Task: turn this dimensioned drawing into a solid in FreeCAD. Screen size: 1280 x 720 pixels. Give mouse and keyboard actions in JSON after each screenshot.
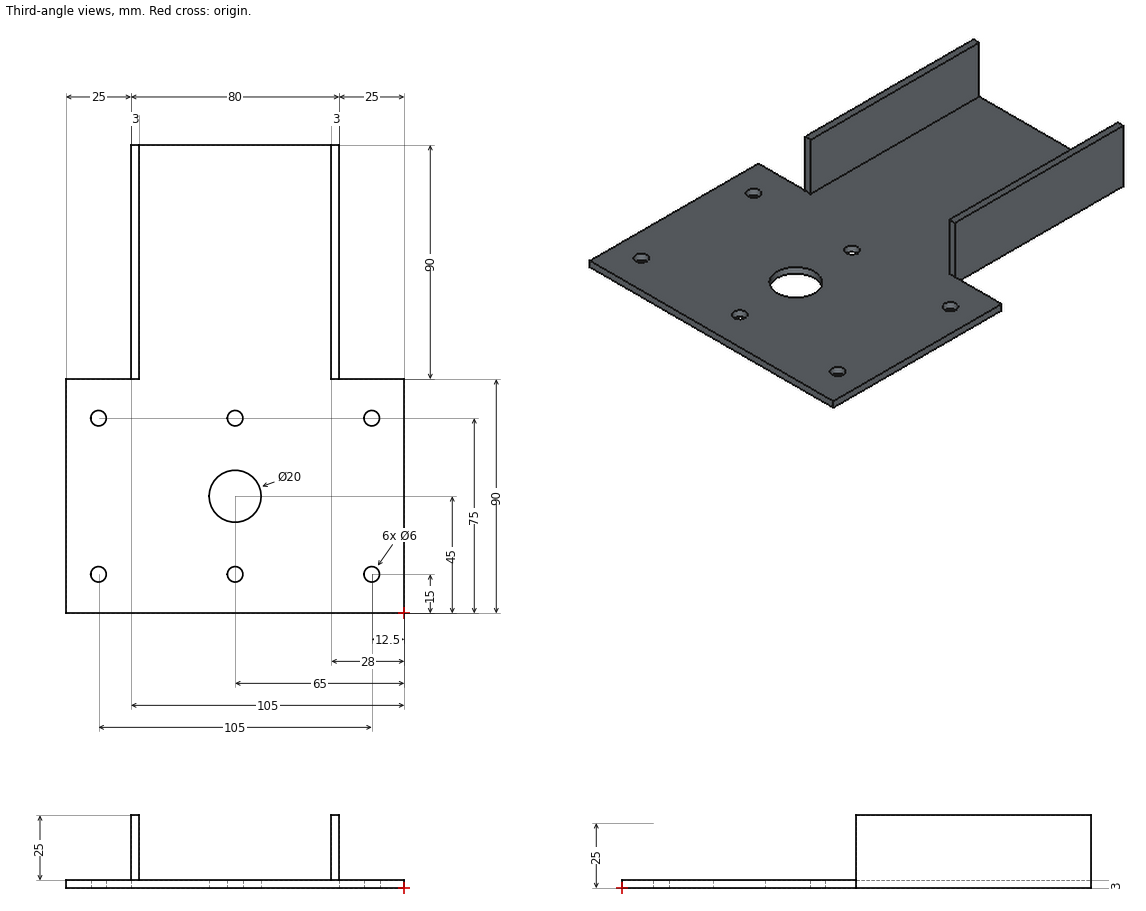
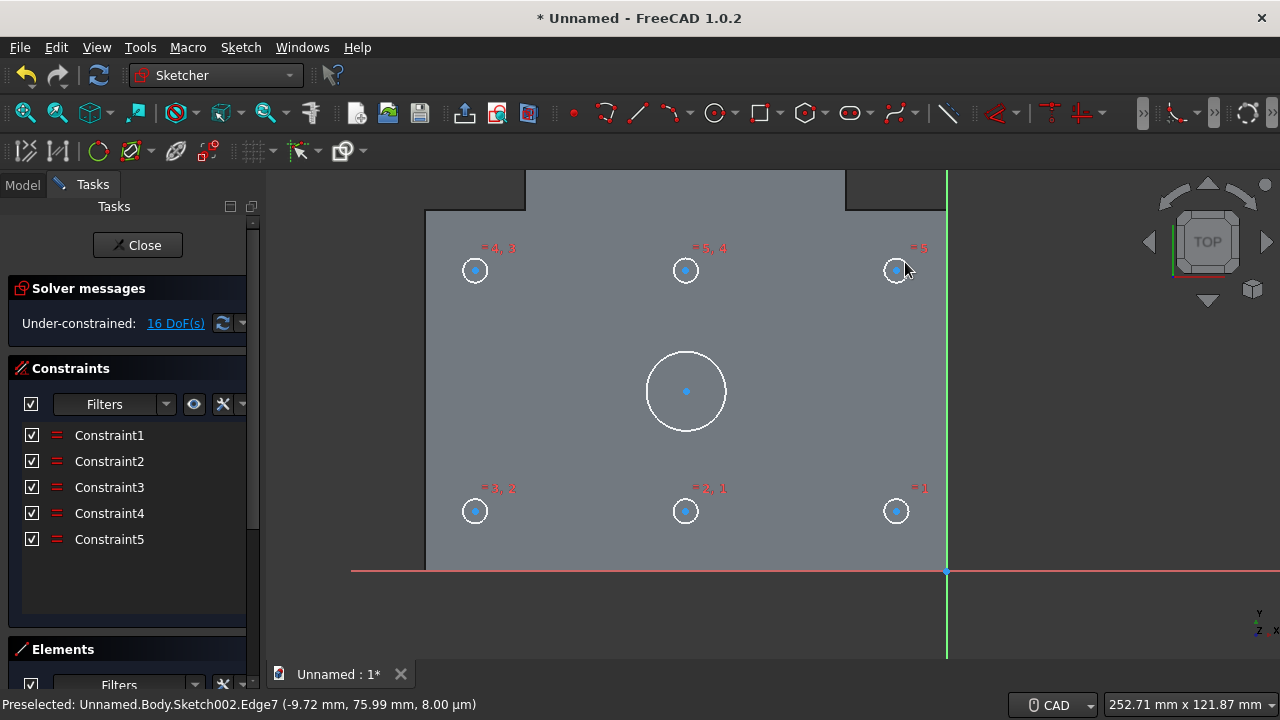
{"action": "left_click", "coordinate": [996, 114]}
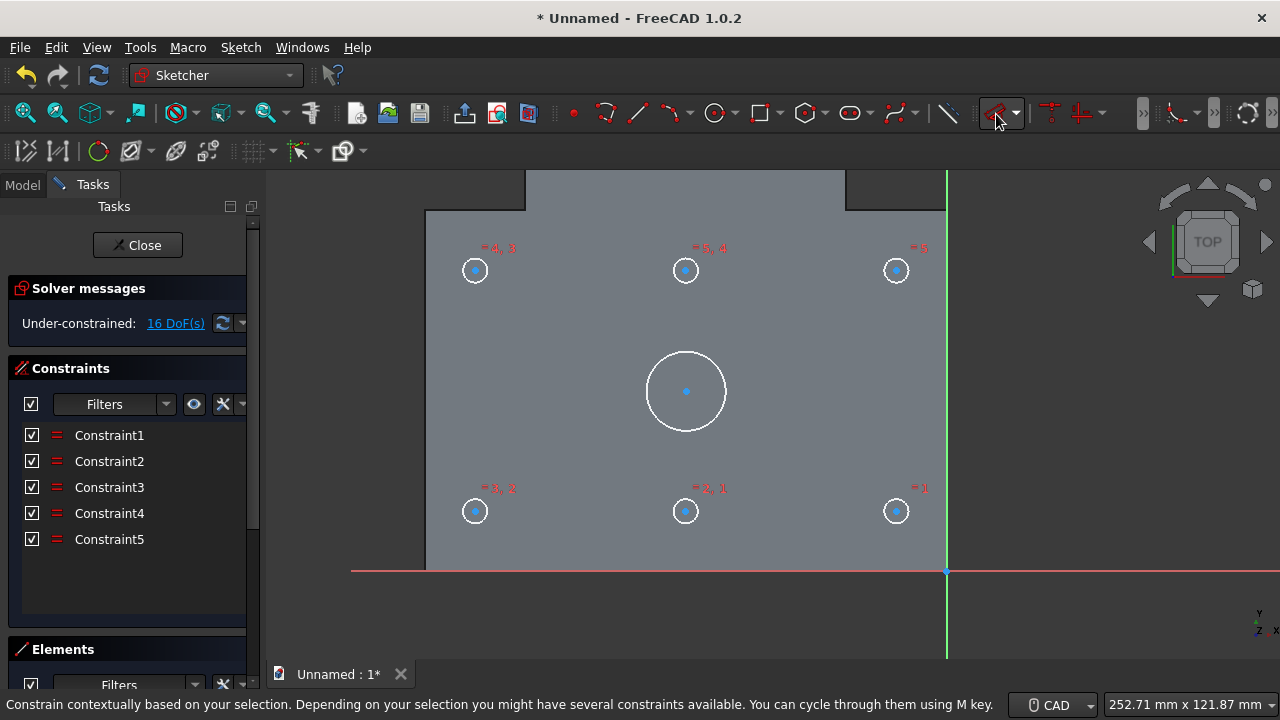
{"action": "left_click", "coordinate": [714, 363]}
{"action": "left_click", "coordinate": [736, 340]}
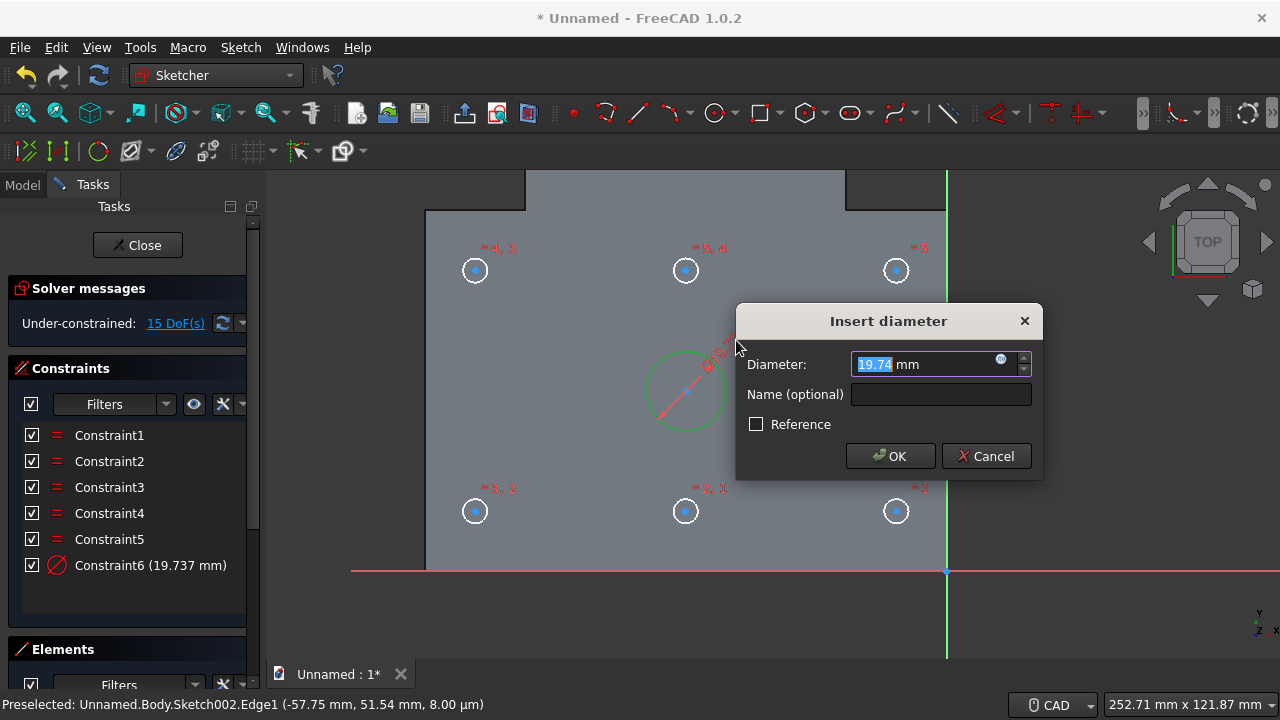
{"action": "type", "text": "20"}
{"action": "key", "text": "Return"}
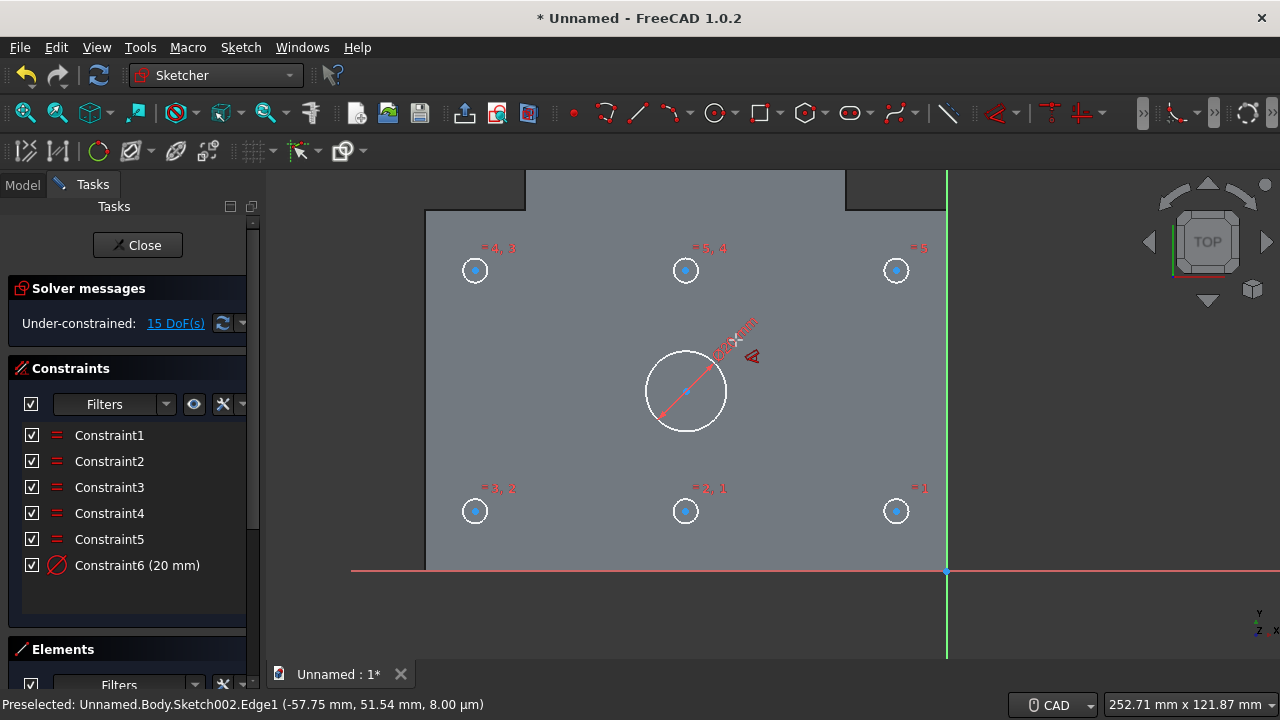
{"action": "scroll", "coordinate": [905, 503], "scroll_direction": "up", "scroll_amount": 3}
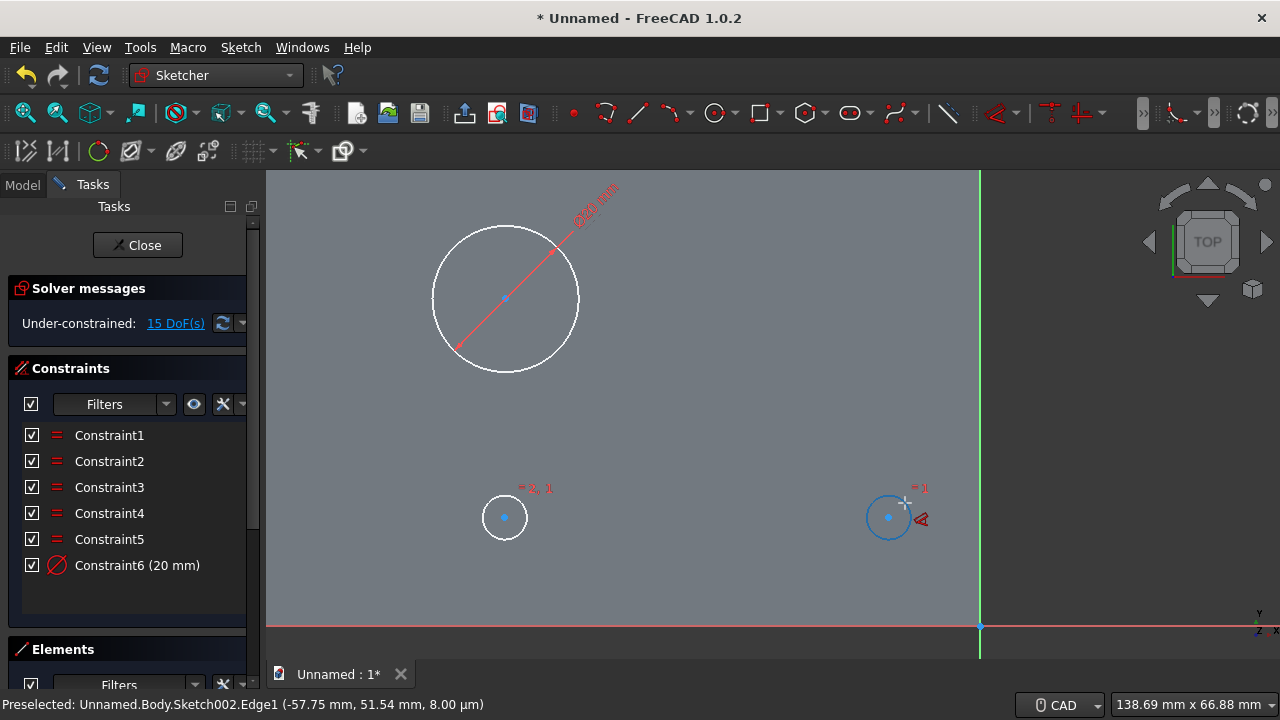
{"action": "left_click", "coordinate": [904, 502]}
{"action": "left_click", "coordinate": [926, 479]}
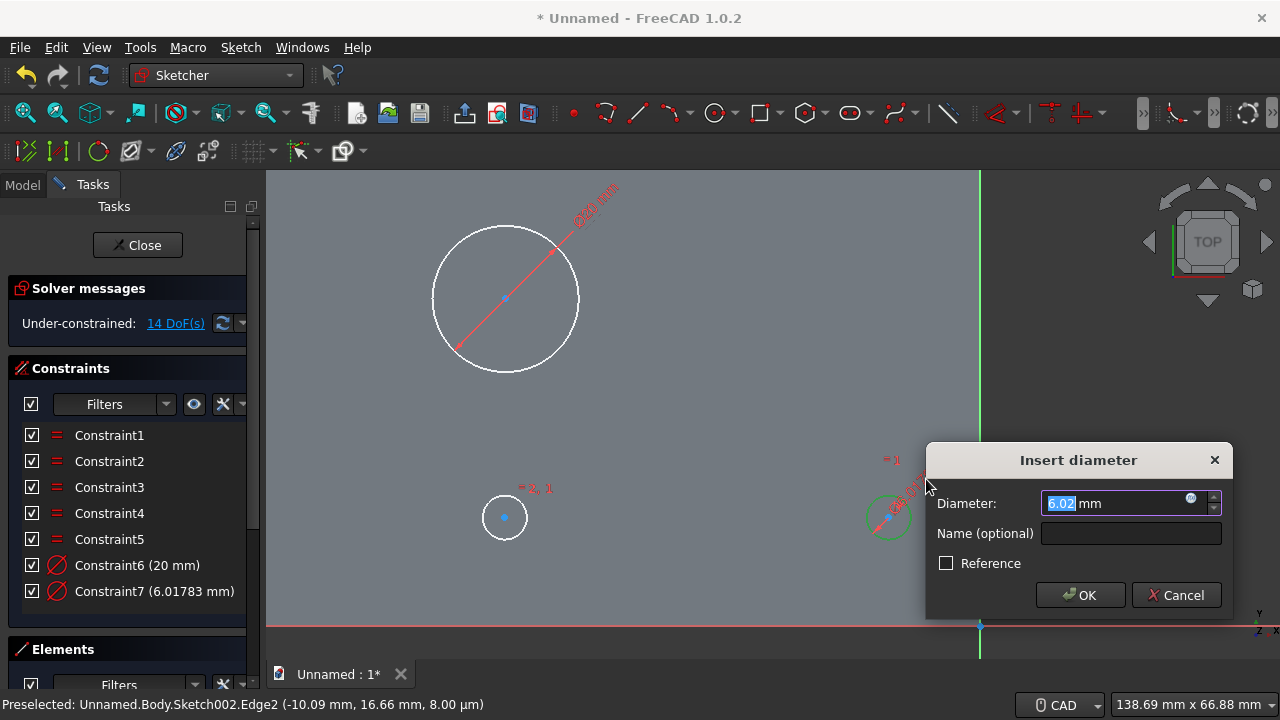
{"action": "type", "text": "6"}
{"action": "key", "text": "Return"}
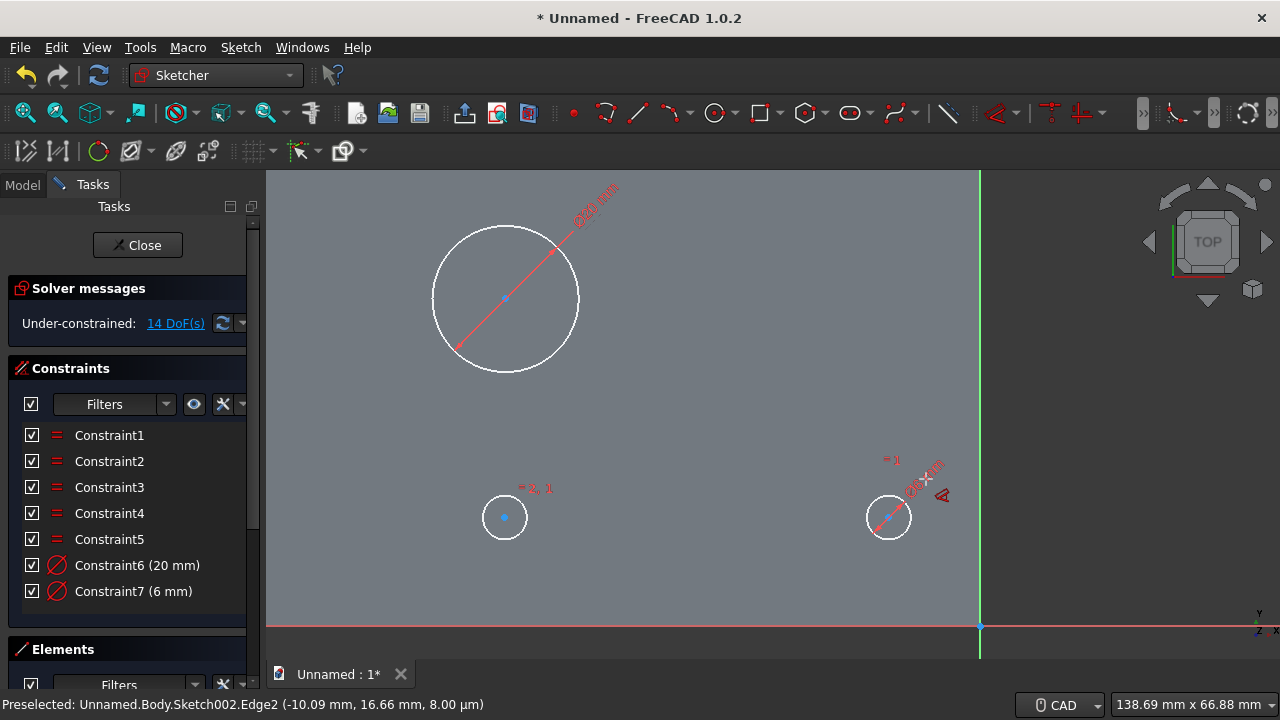
{"action": "left_click", "coordinate": [506, 299]}
{"action": "left_click", "coordinate": [743, 265]}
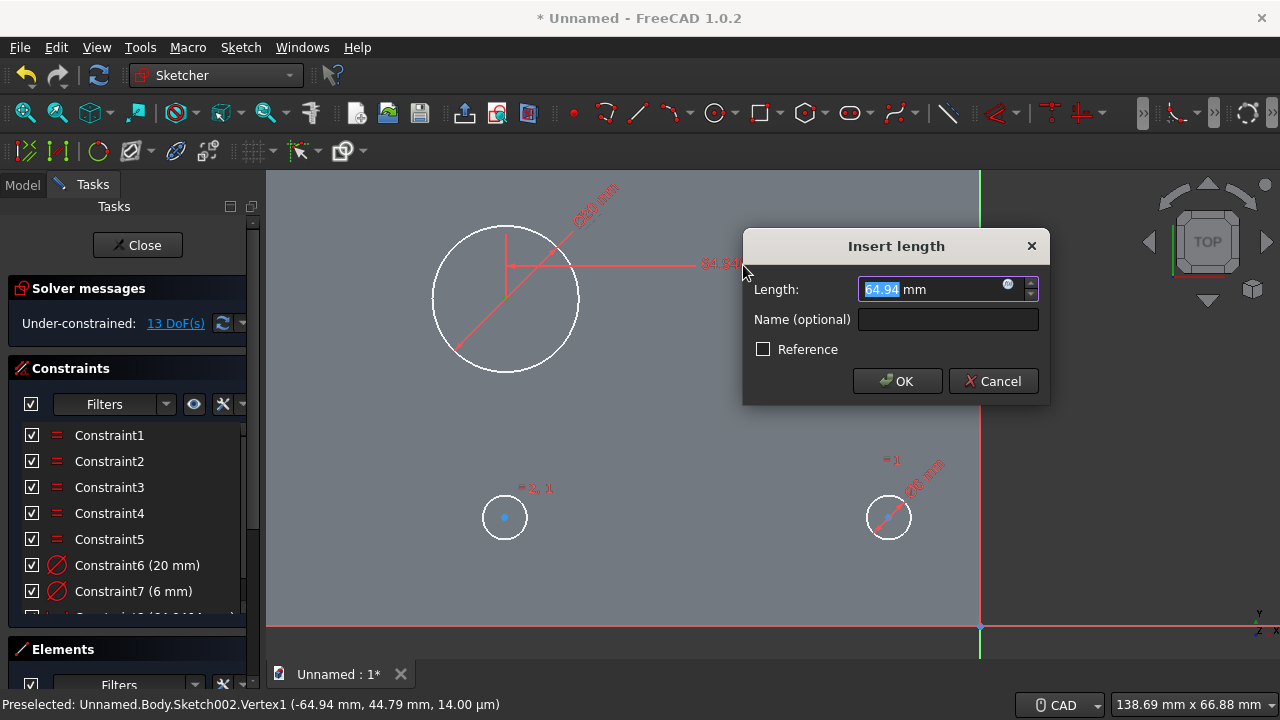
{"action": "type", "text": "65"}
{"action": "key", "text": "Return"}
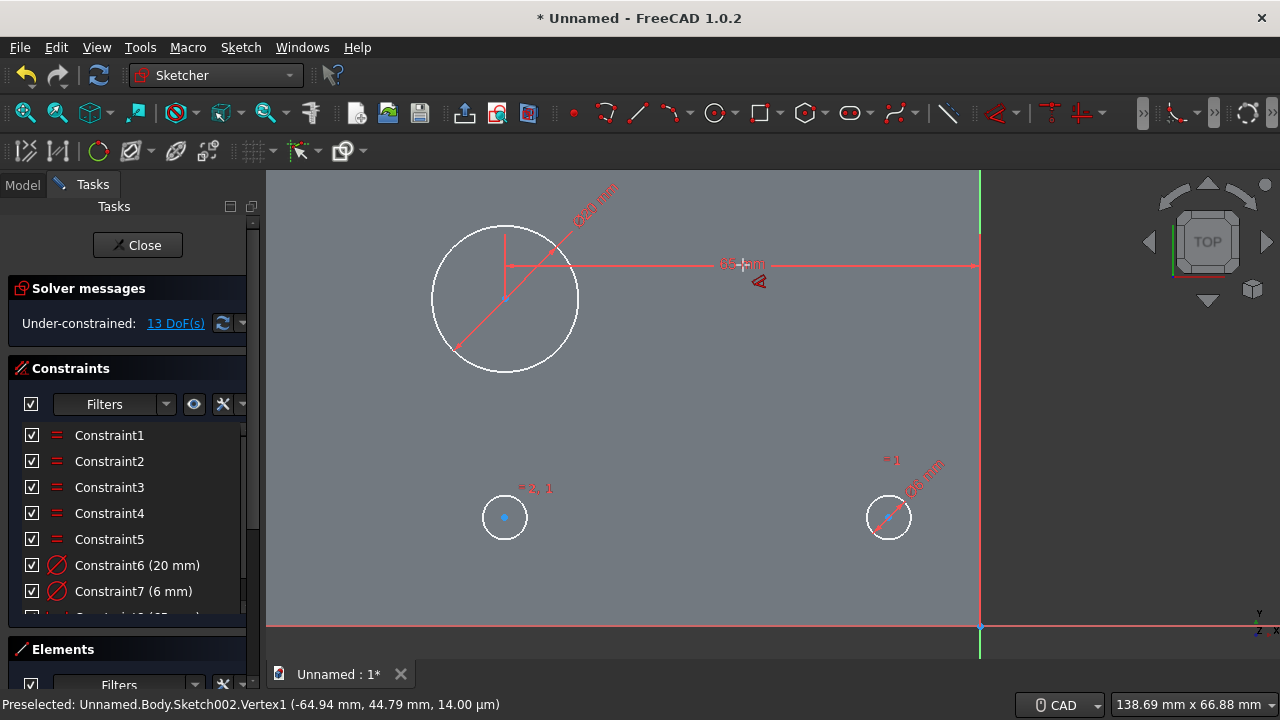
{"action": "left_click", "coordinate": [505, 299]}
{"action": "left_click", "coordinate": [1014, 463]}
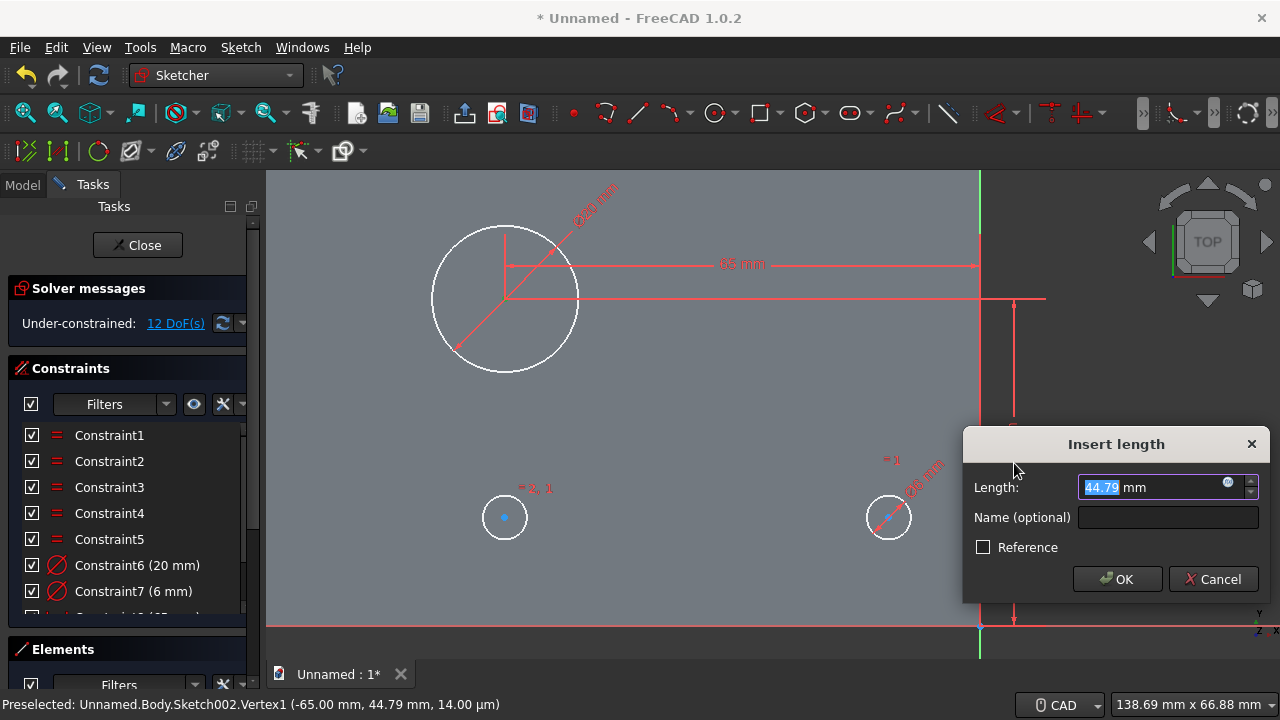
{"action": "type", "text": "45"}
{"action": "key", "text": "Return"}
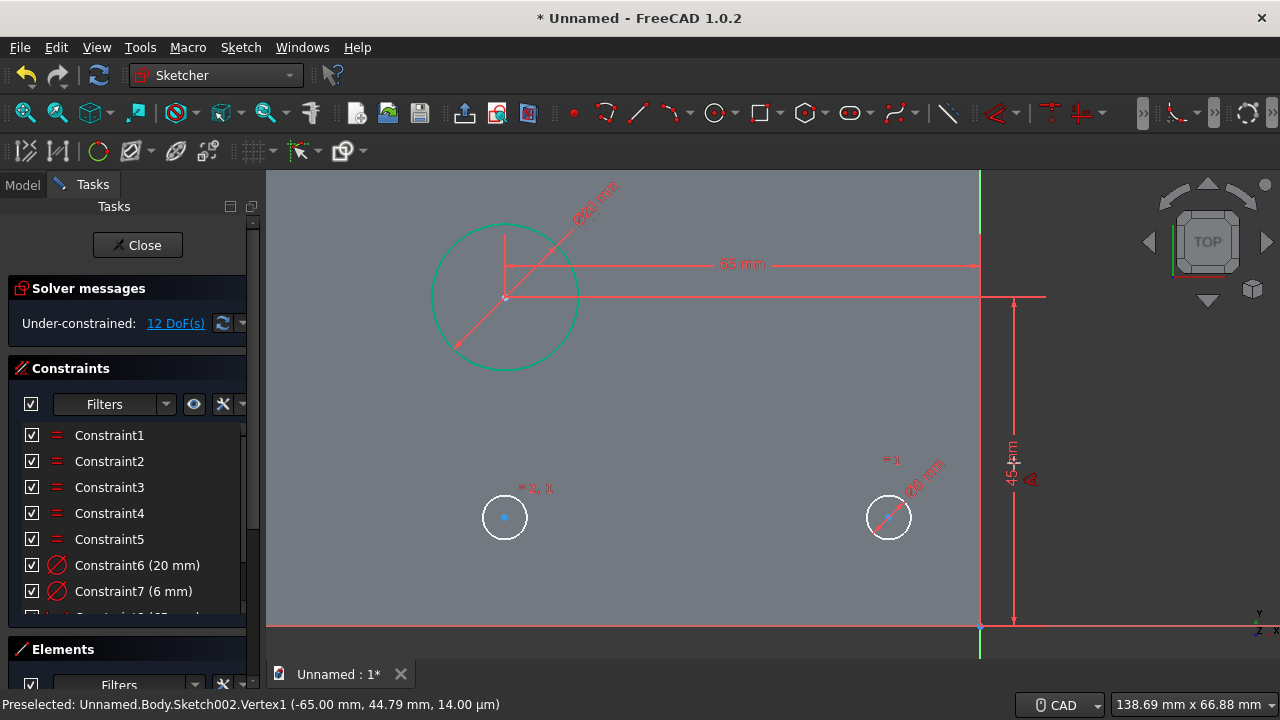
{"action": "left_click", "coordinate": [889, 518]}
{"action": "left_click", "coordinate": [1014, 572]}